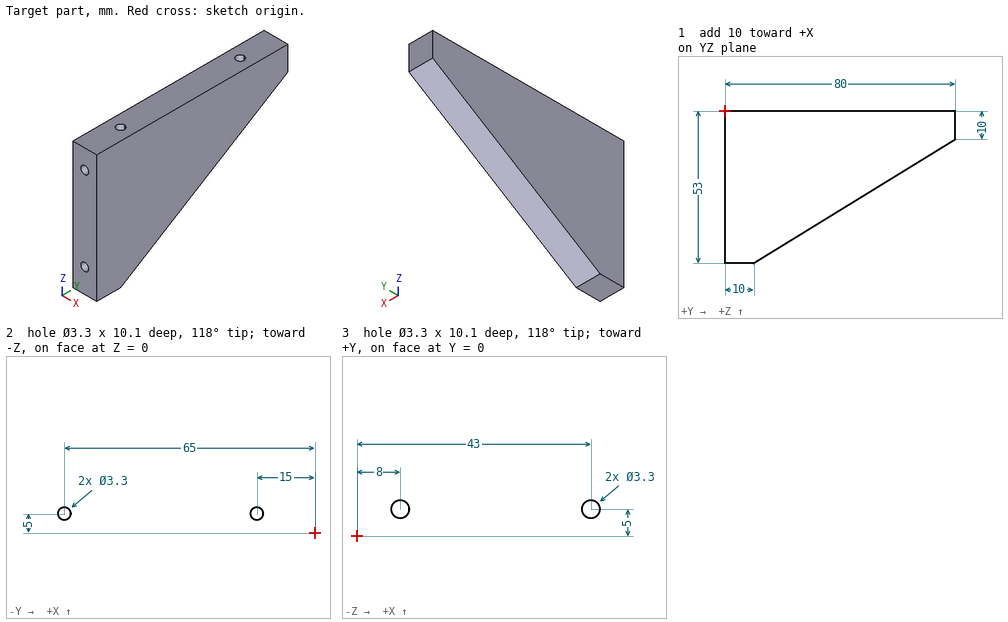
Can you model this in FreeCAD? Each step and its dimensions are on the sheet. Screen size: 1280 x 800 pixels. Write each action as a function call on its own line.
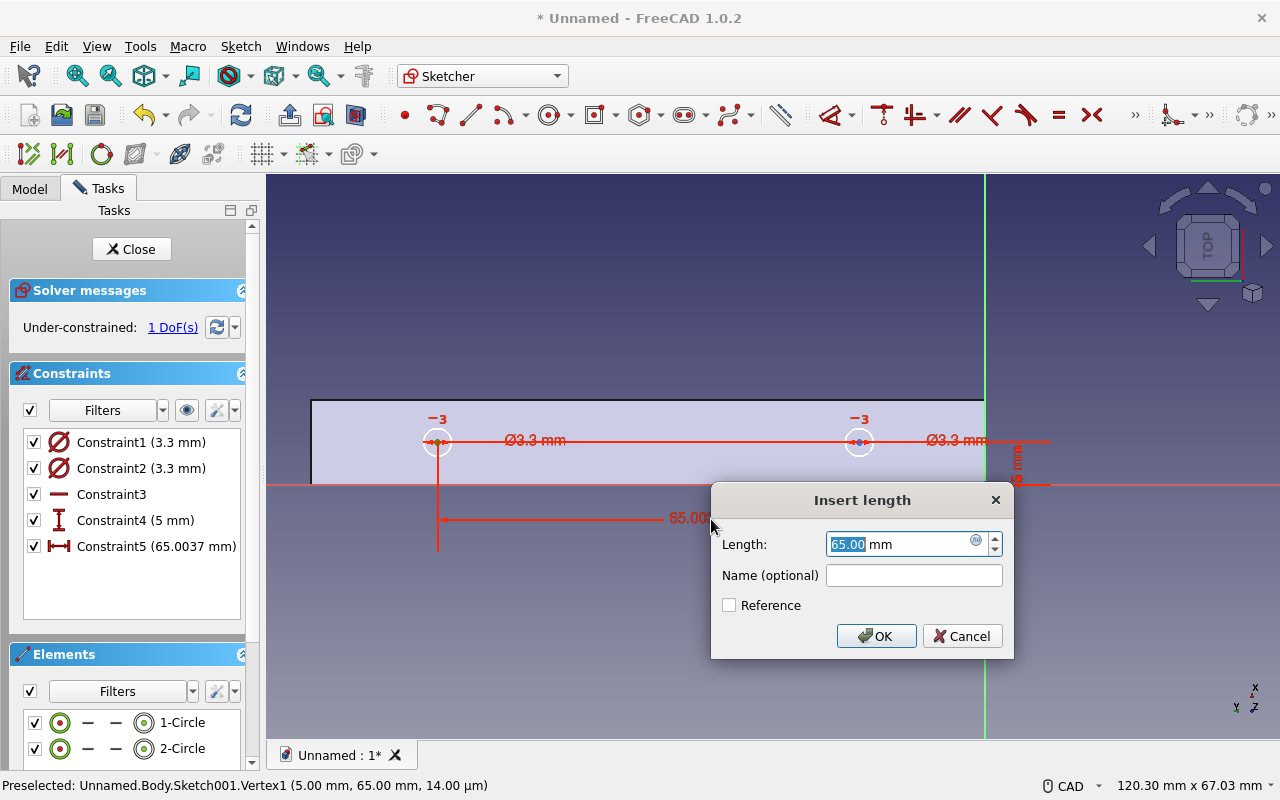
text(65)
key(Return)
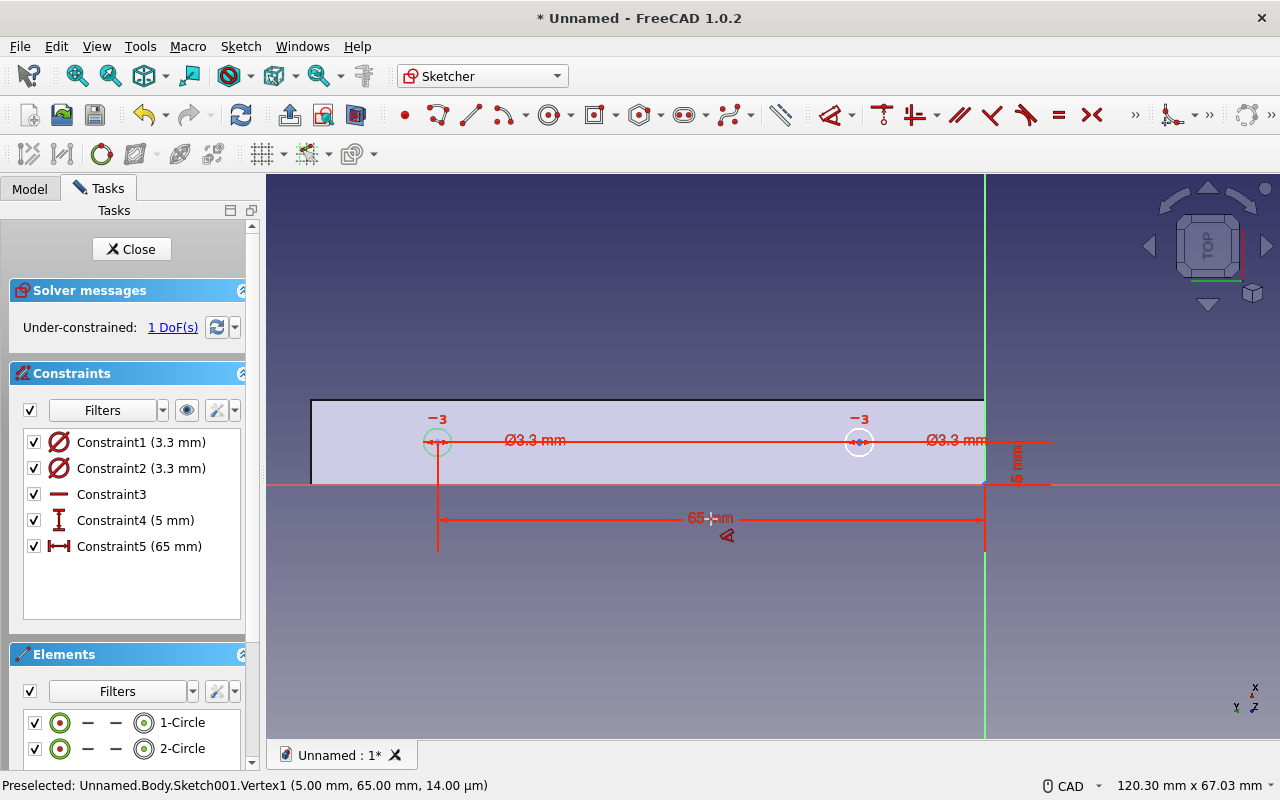
click(859, 442)
click(922, 519)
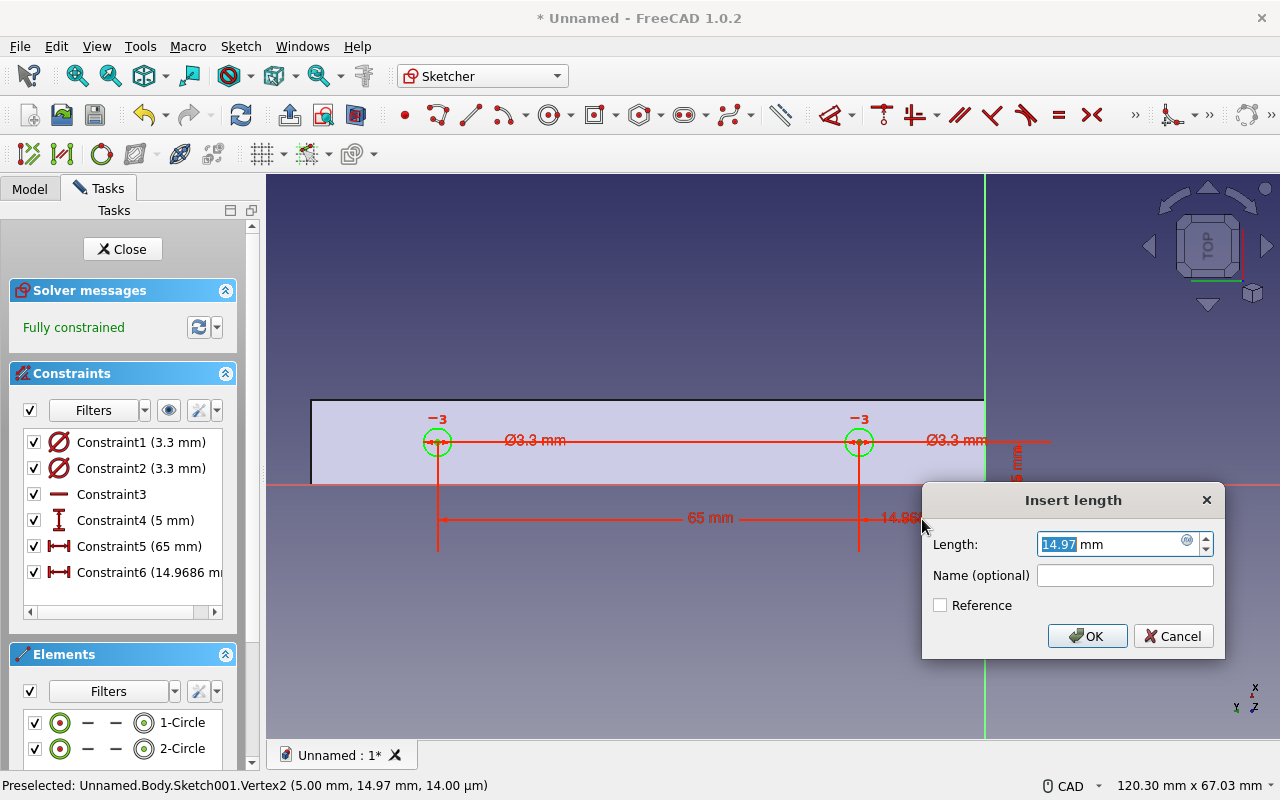
text(15)
key(Return)
key(Escape)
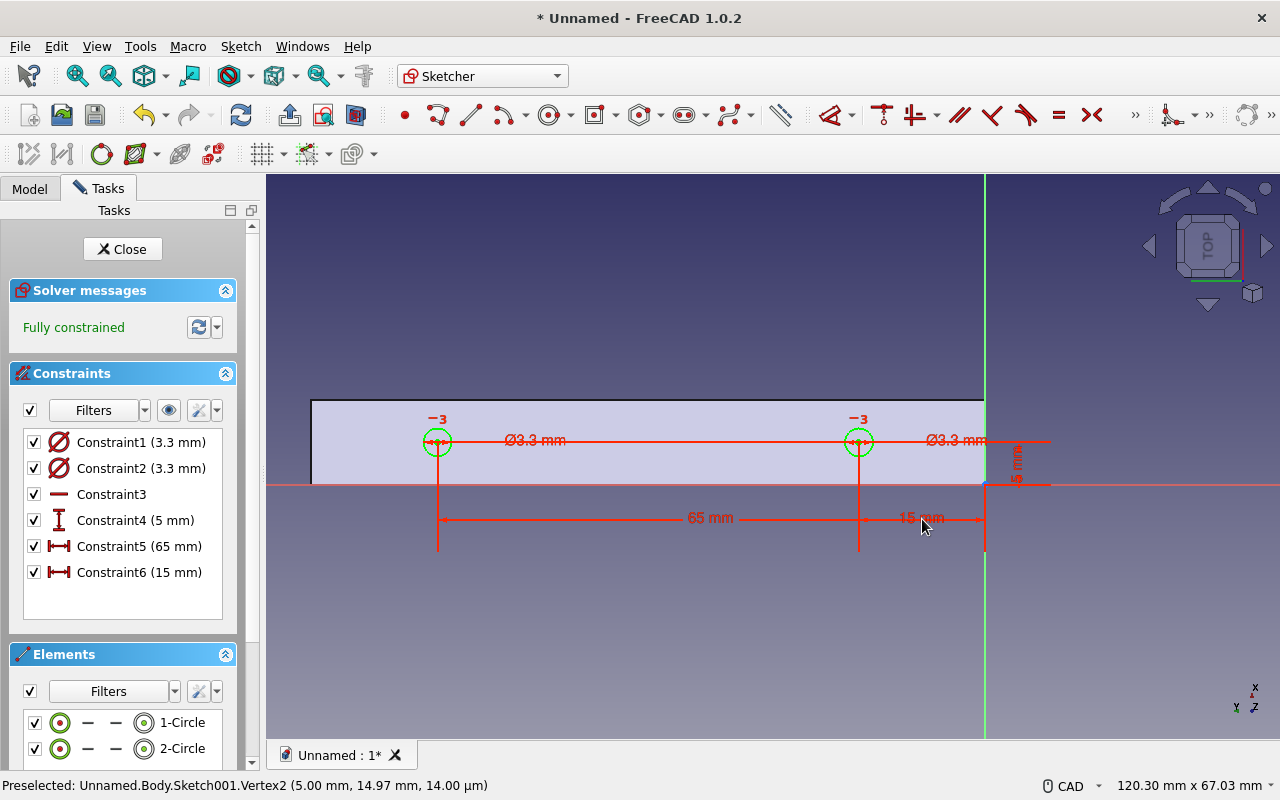
click(123, 249)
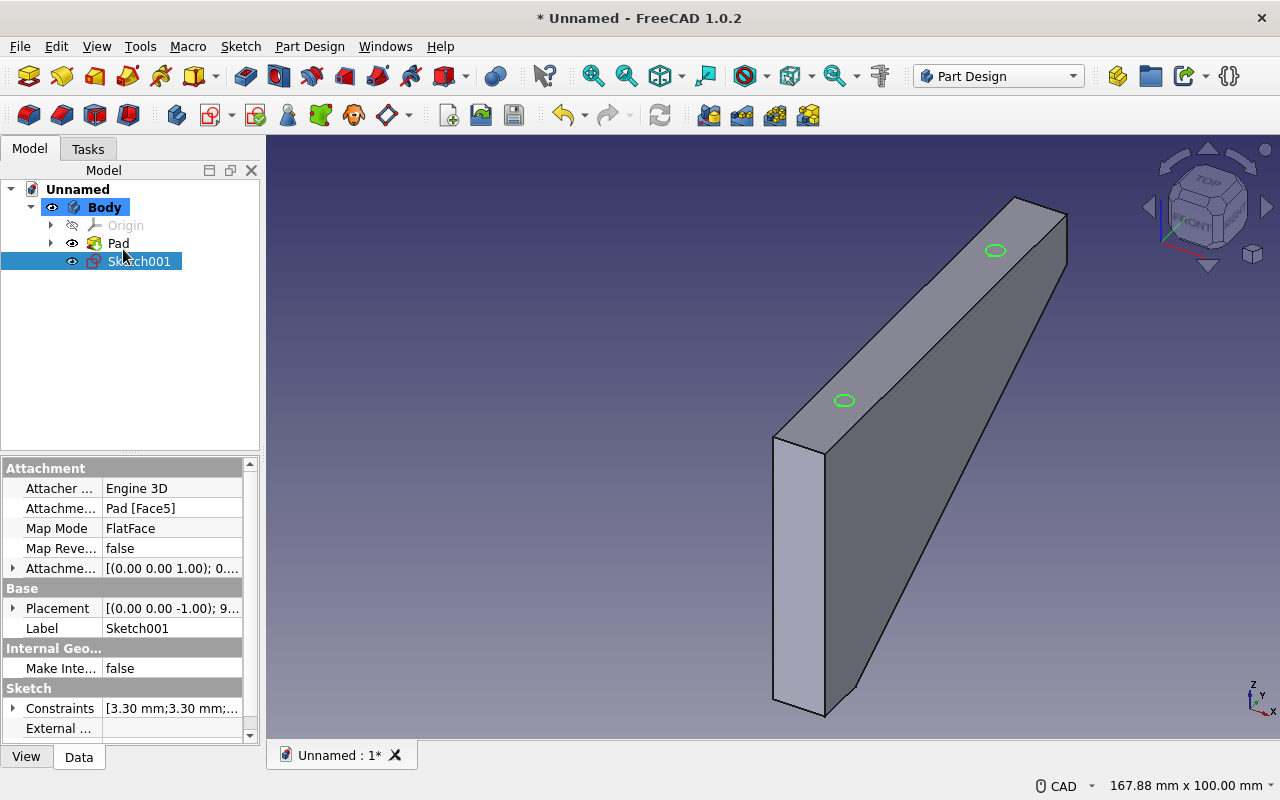
click(279, 76)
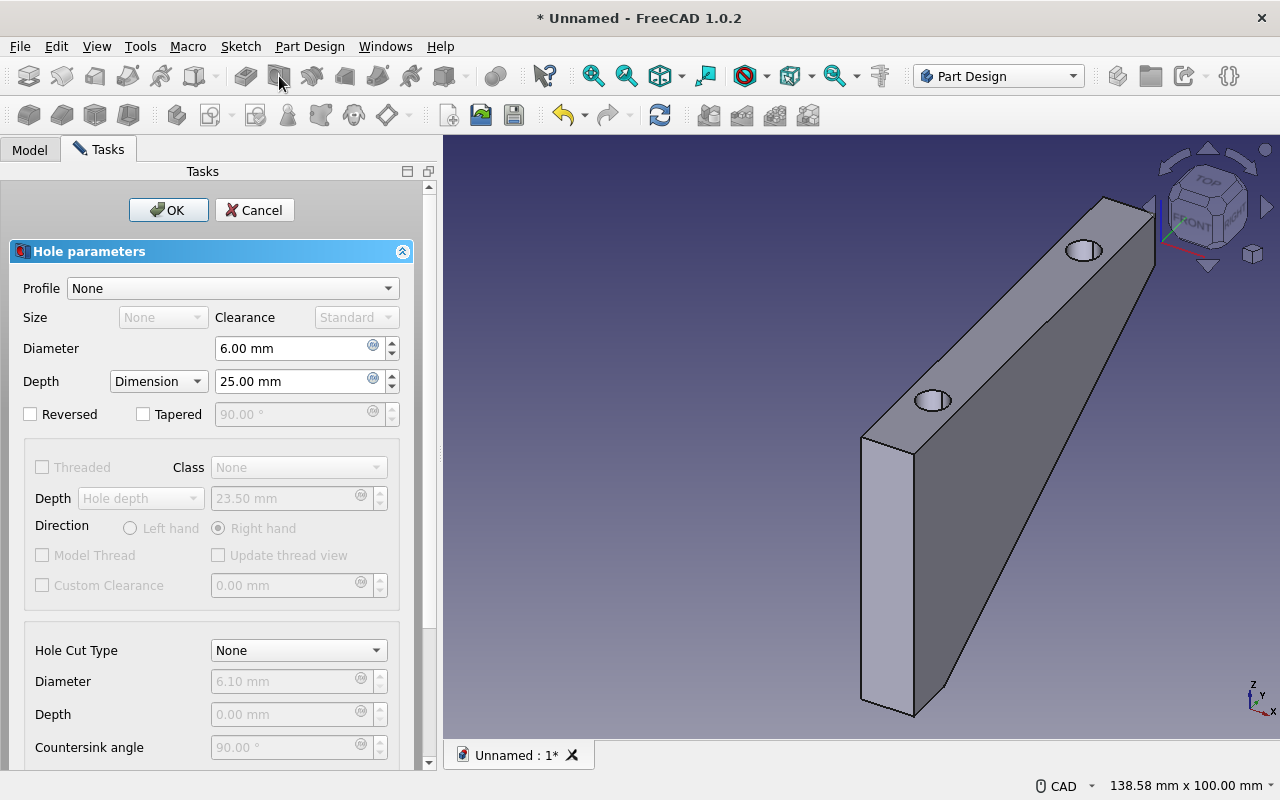
triple_click(300, 348)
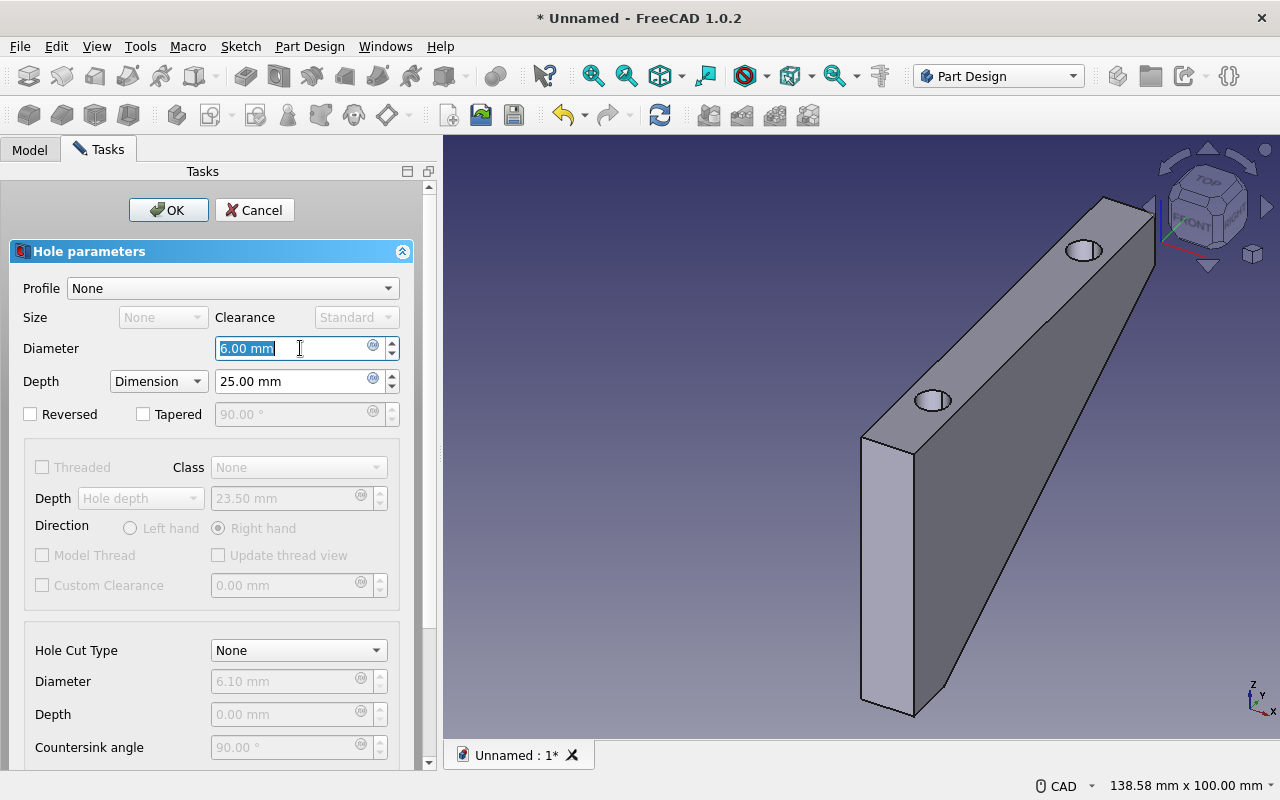
text(3.3)
key(Tab)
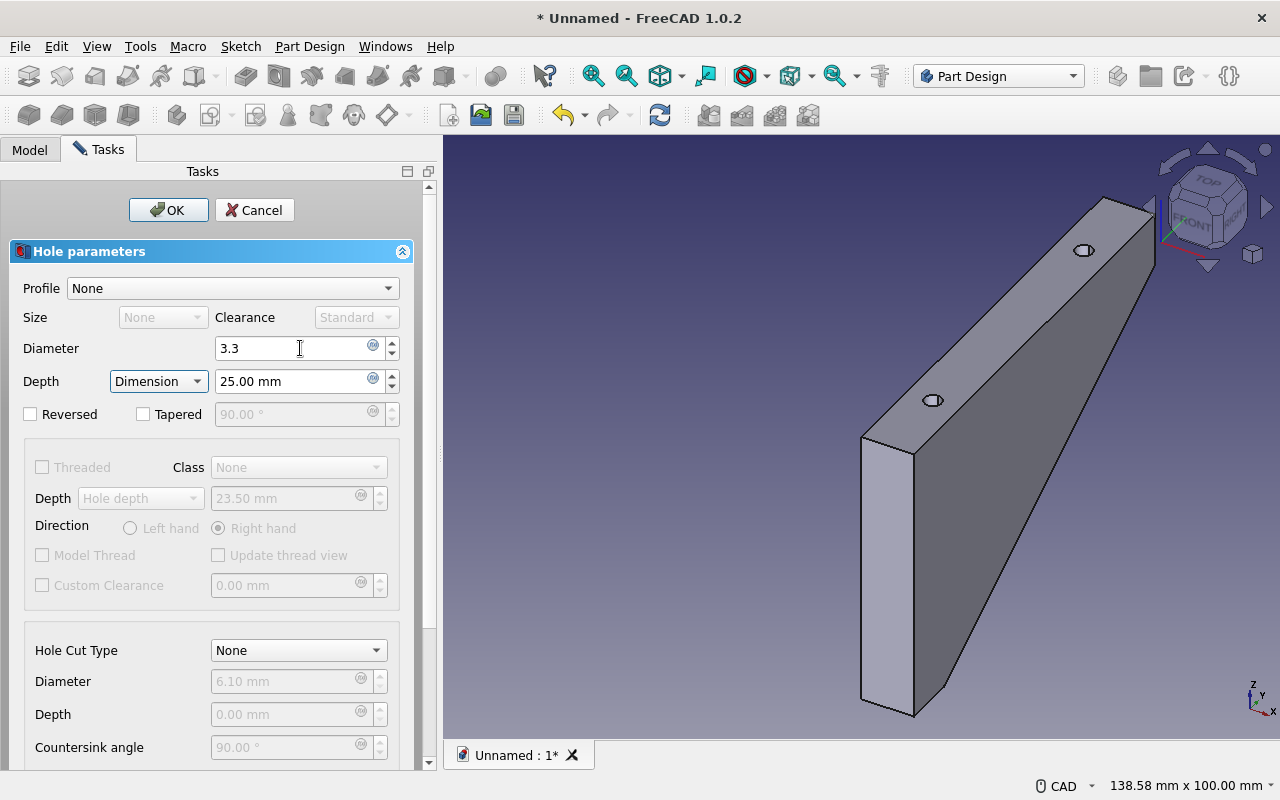
triple_click(300, 382)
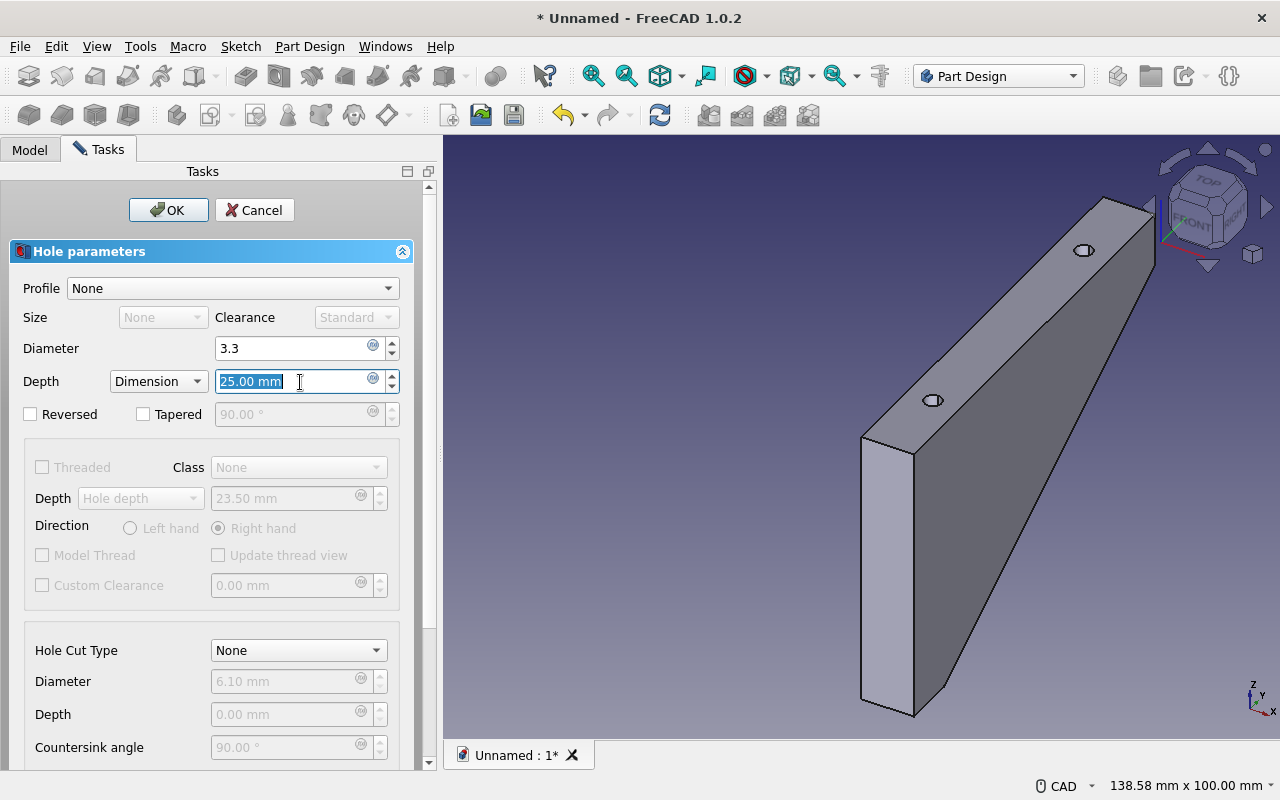
text(10.1)
key(Tab)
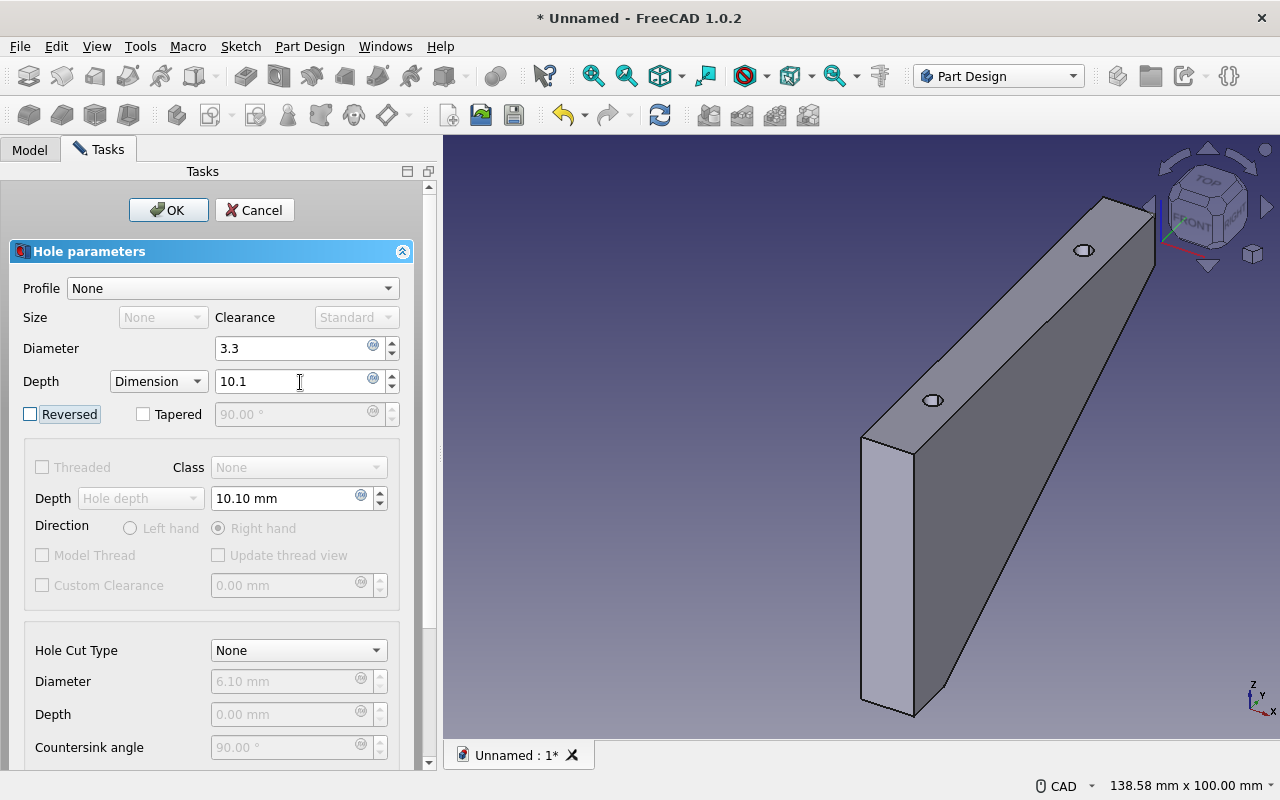
click(169, 210)